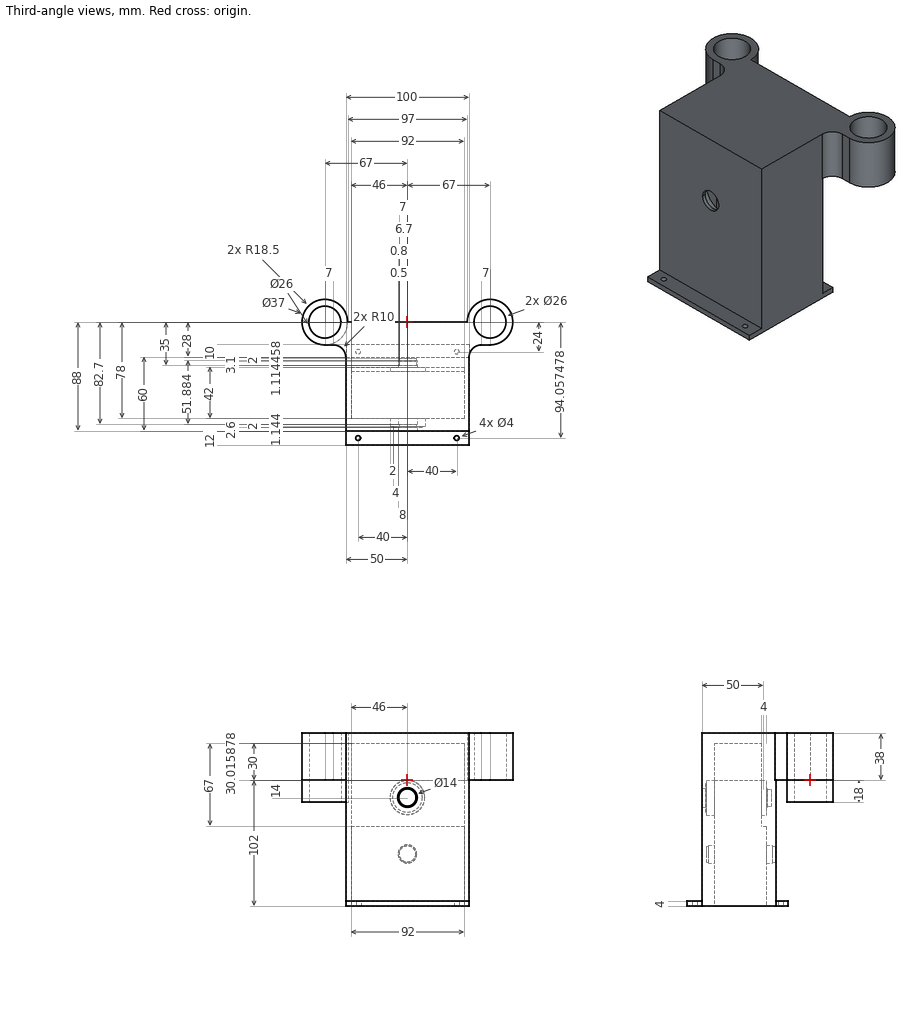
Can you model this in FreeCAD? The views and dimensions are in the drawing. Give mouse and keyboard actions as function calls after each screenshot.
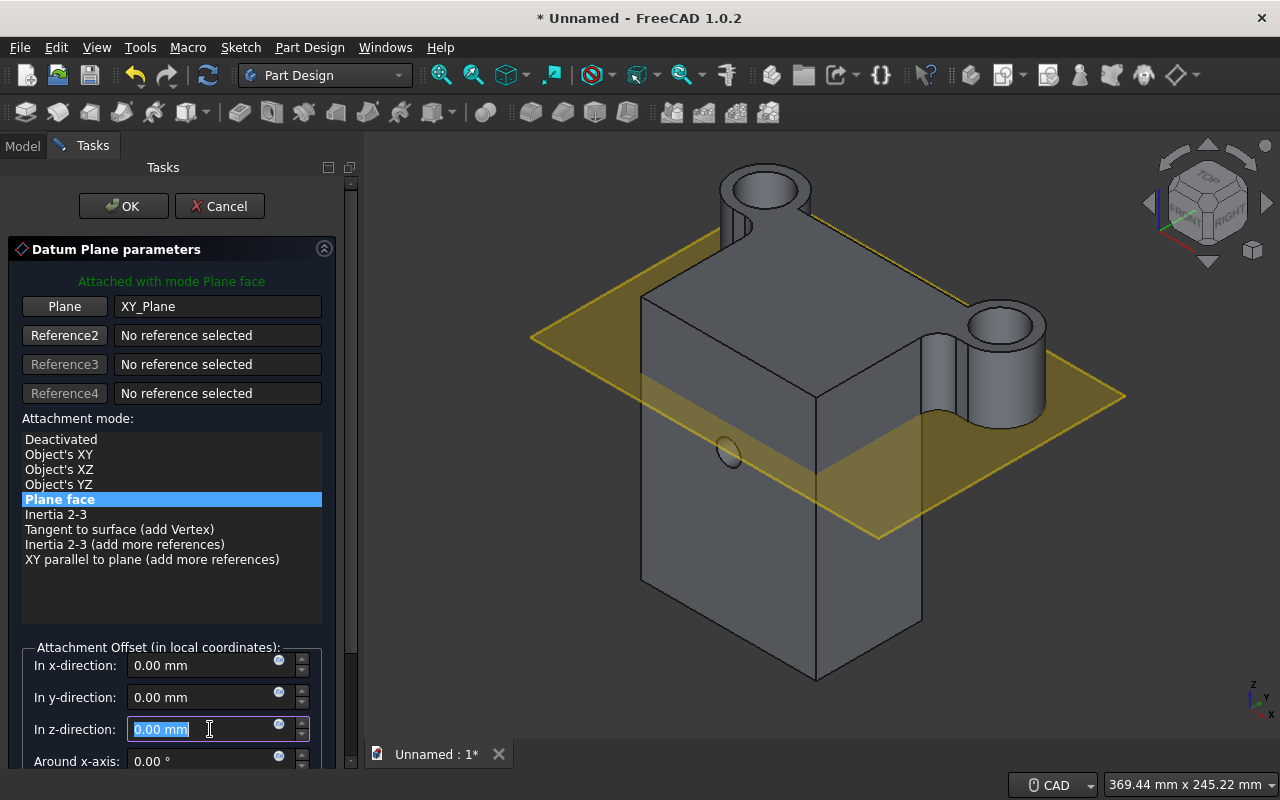
text(-18)
key(Tab)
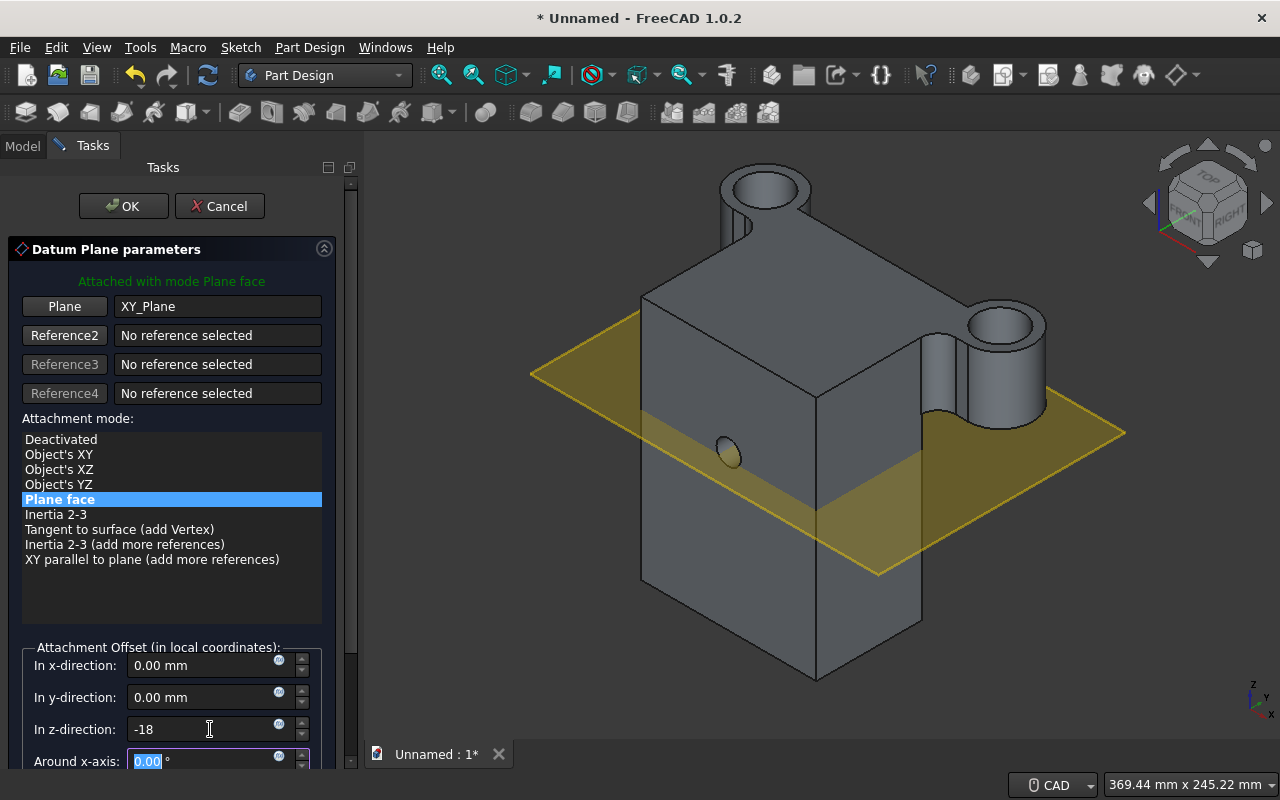
click(124, 206)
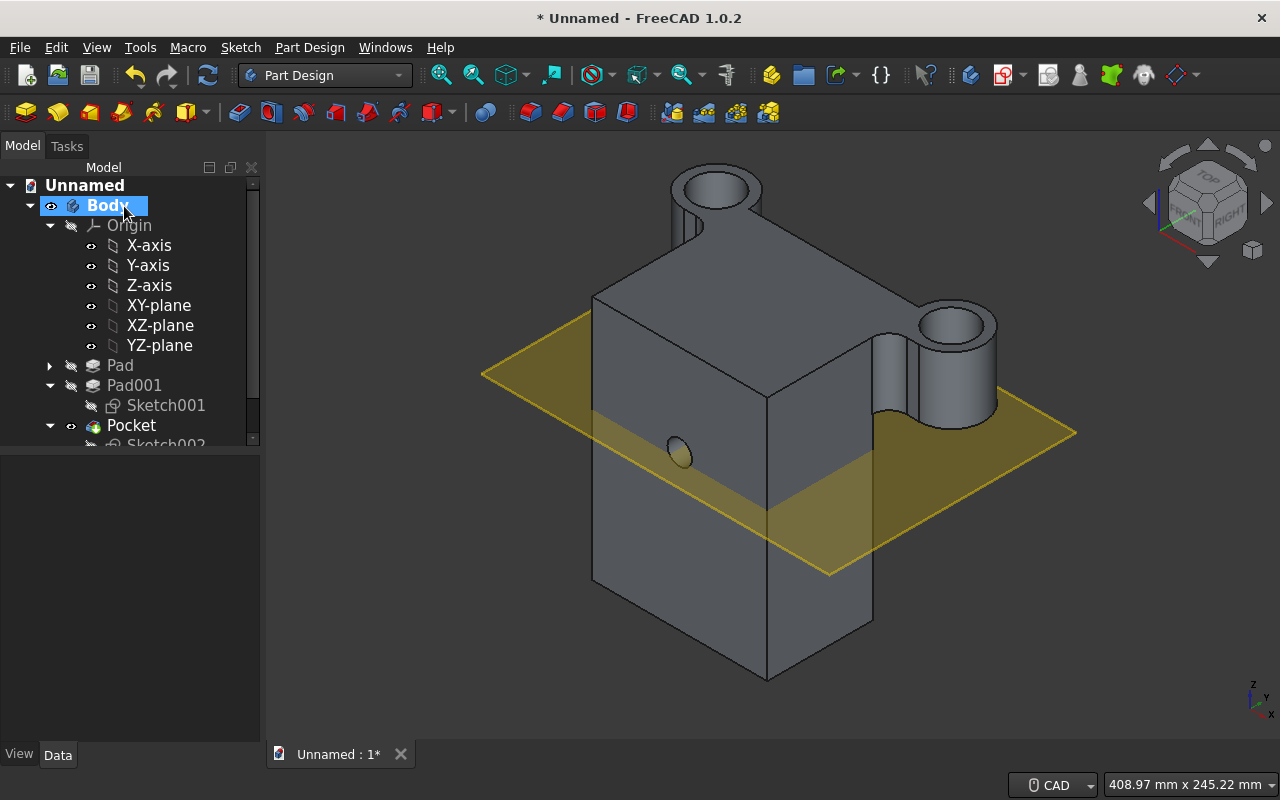
scroll(100, 321, down, 3)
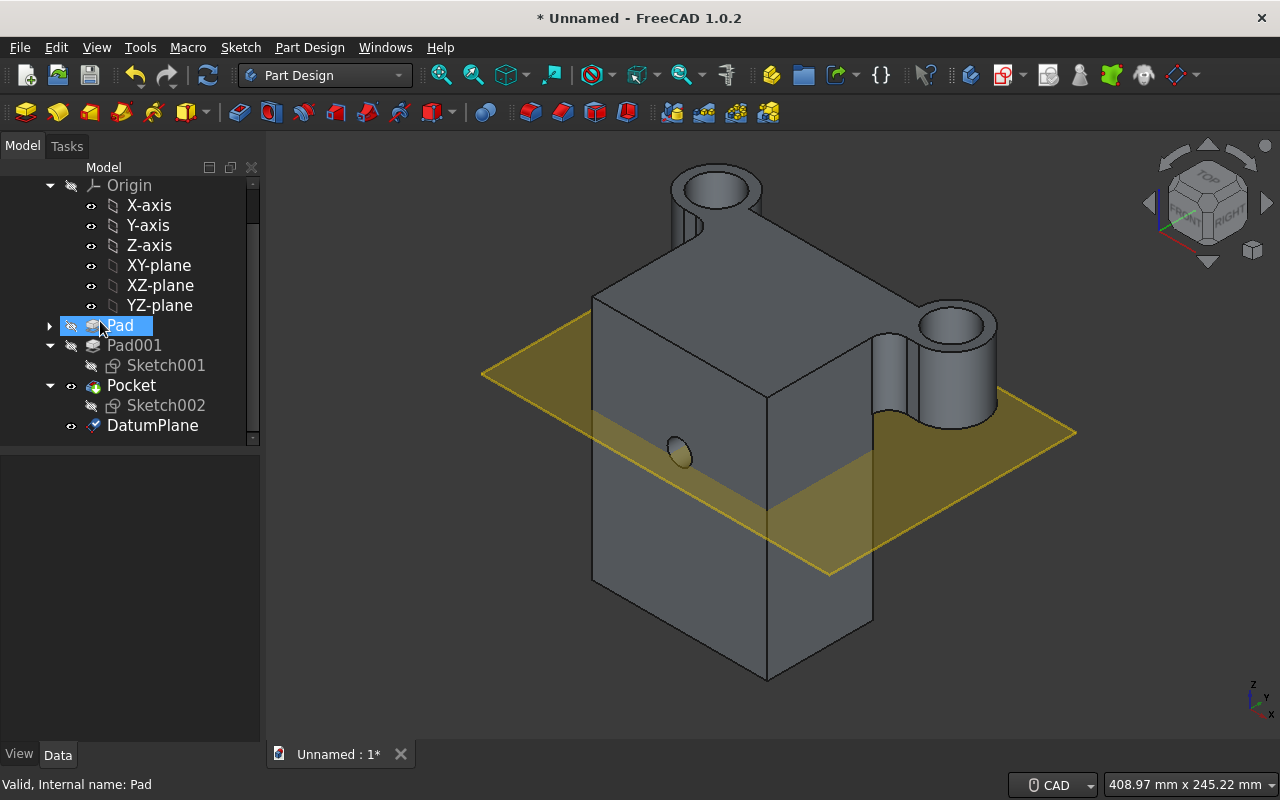
click(116, 426)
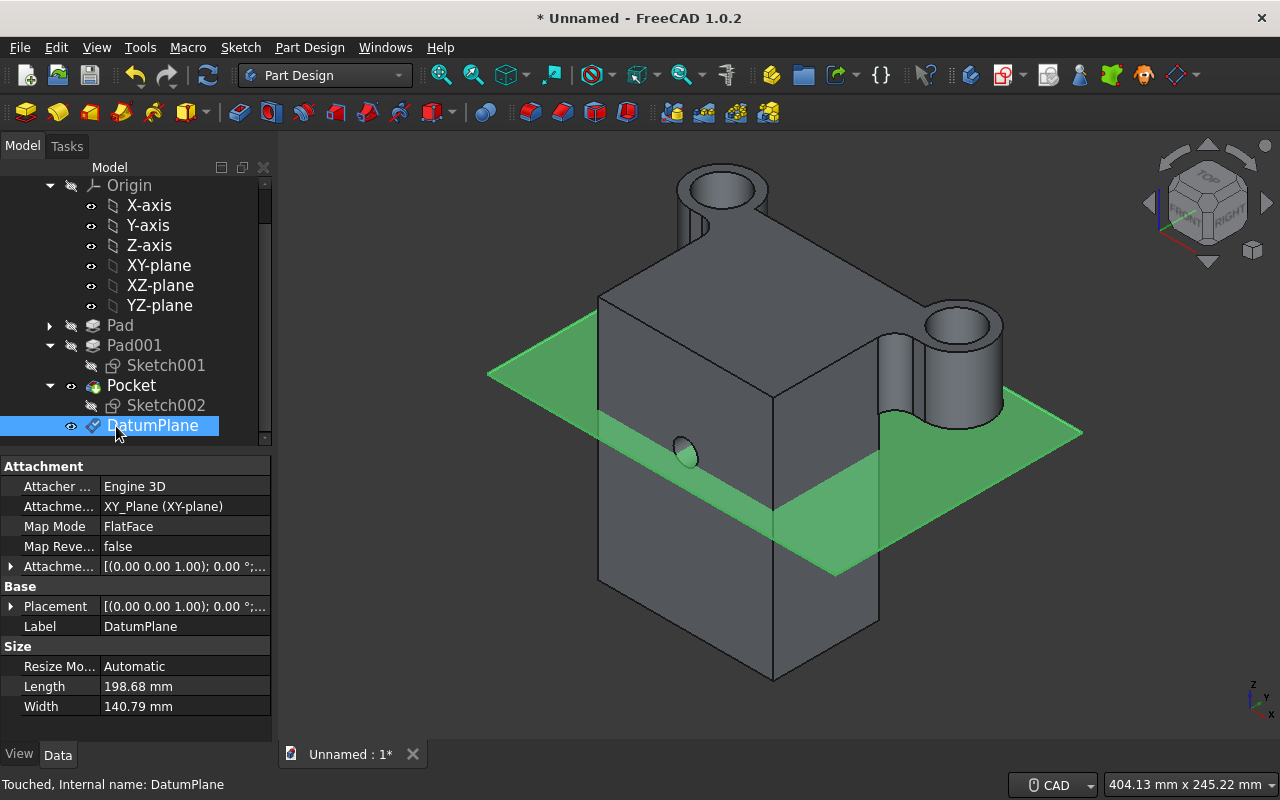
click(1004, 76)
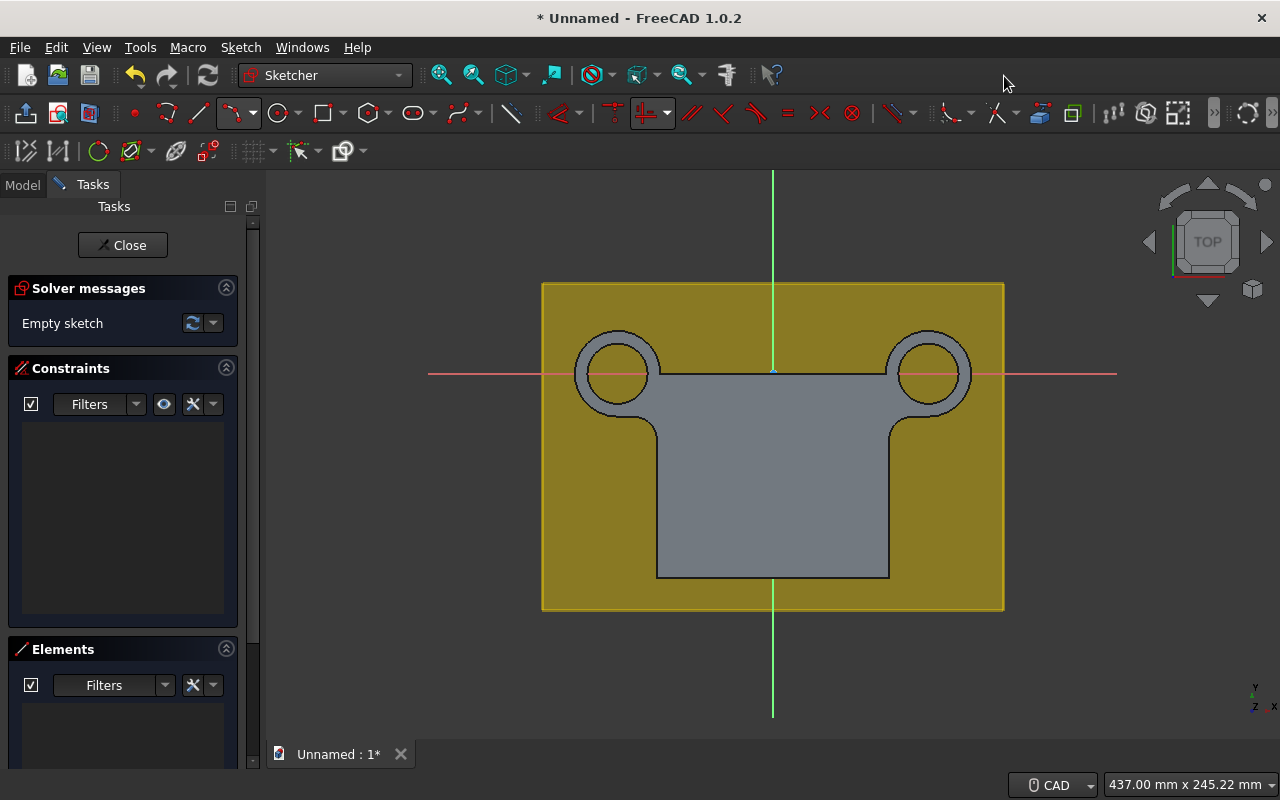
key(q)
key(s)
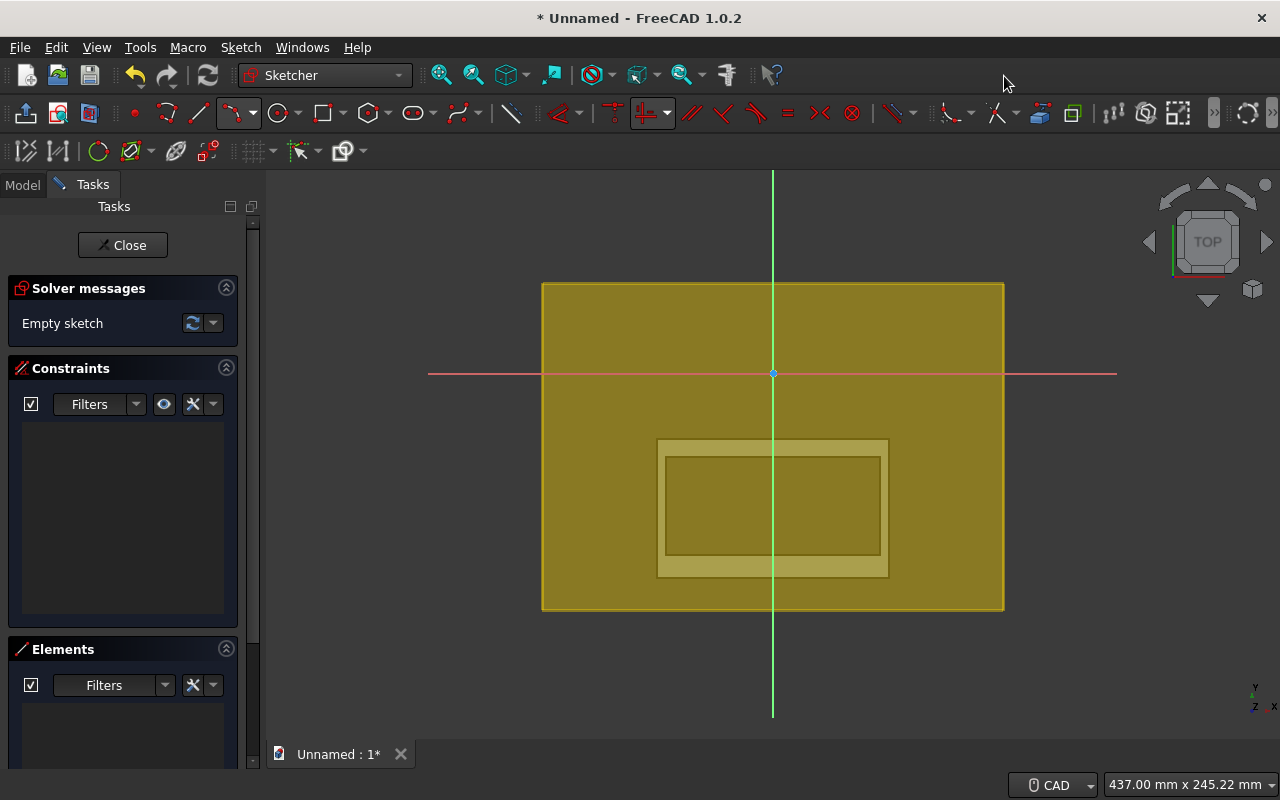
scroll(656, 327, up, 5)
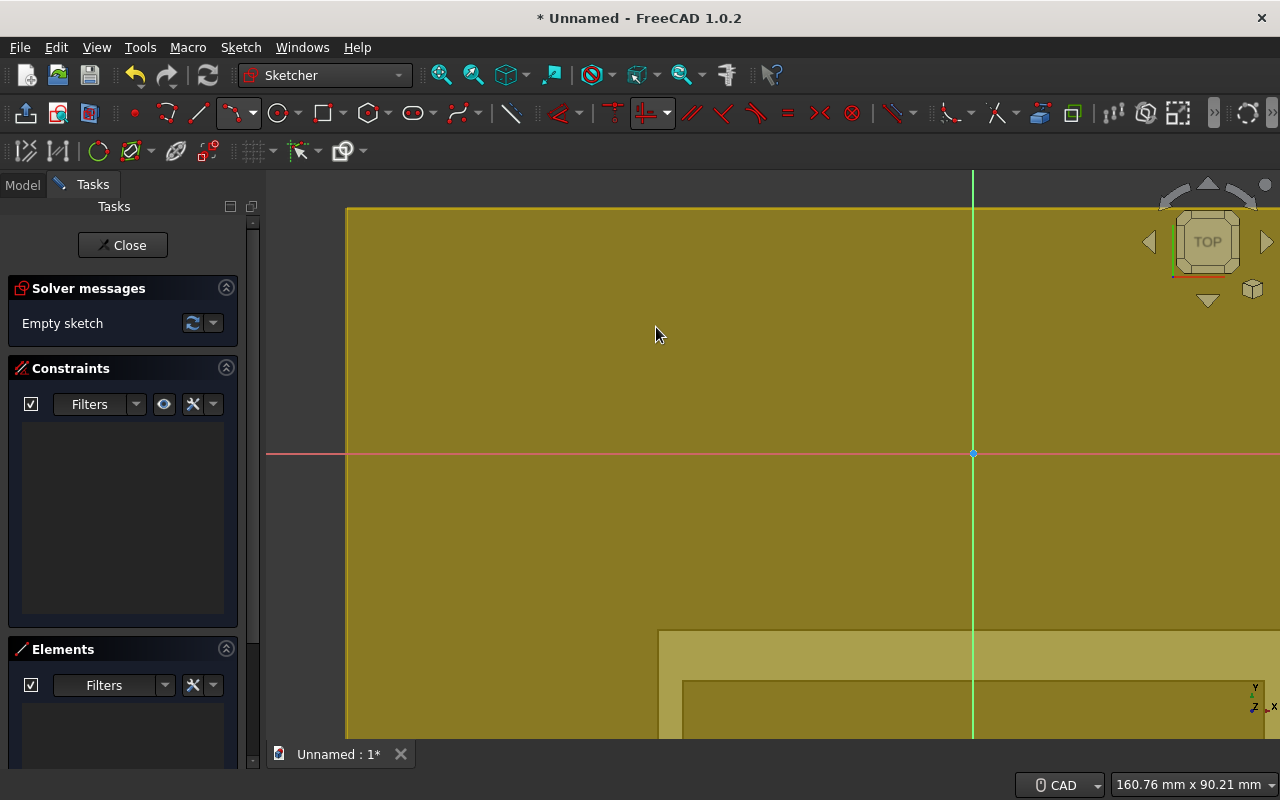
key(g)
key(c)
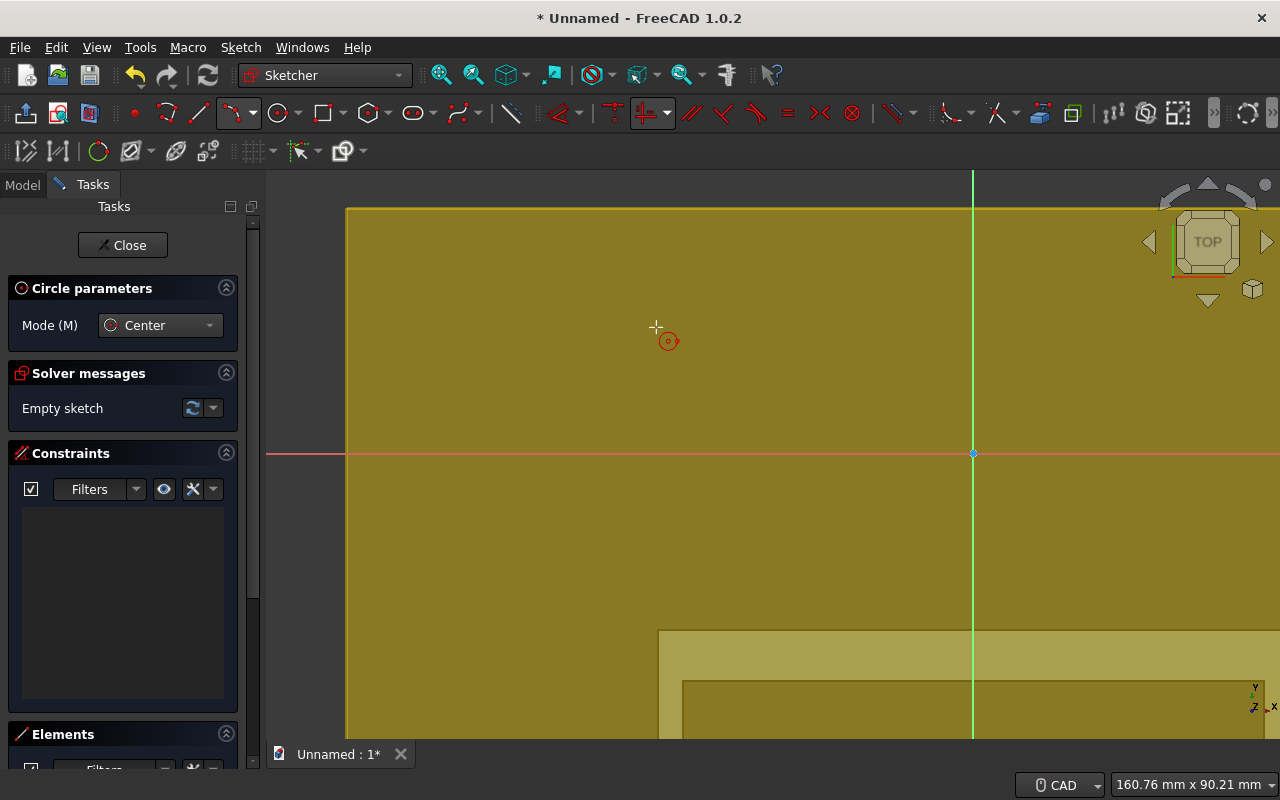
click(551, 454)
click(633, 371)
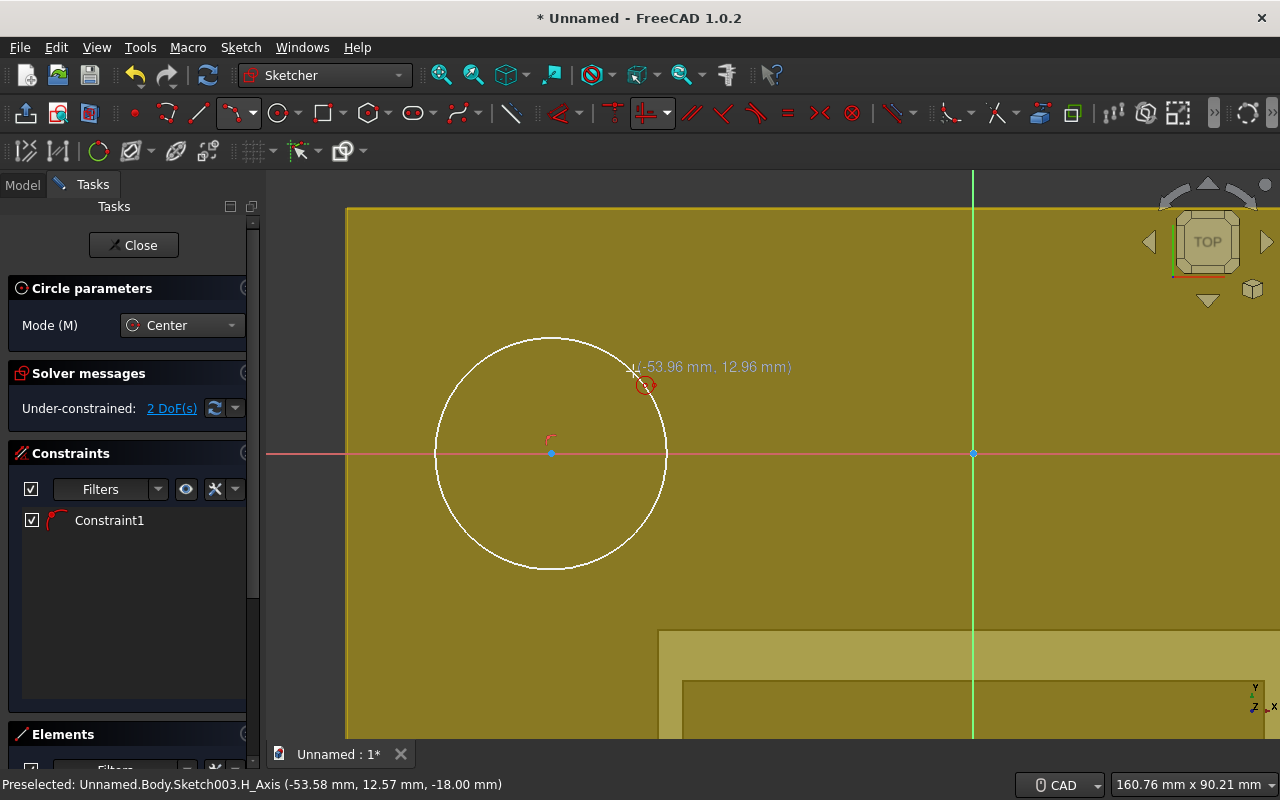
click(551, 454)
click(609, 396)
key(Escape)